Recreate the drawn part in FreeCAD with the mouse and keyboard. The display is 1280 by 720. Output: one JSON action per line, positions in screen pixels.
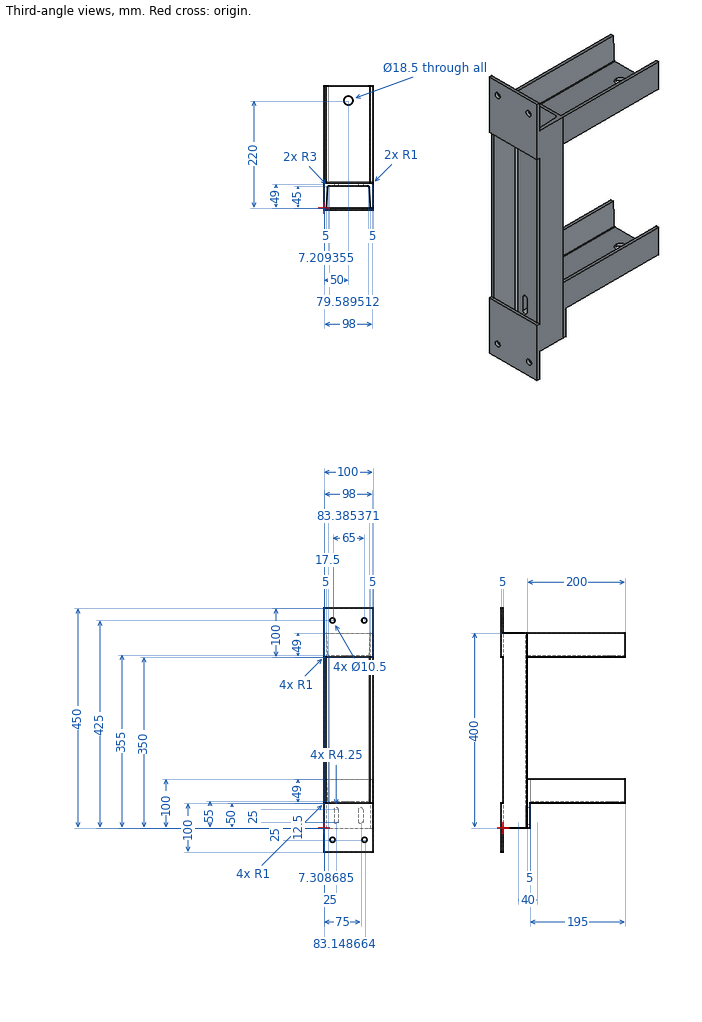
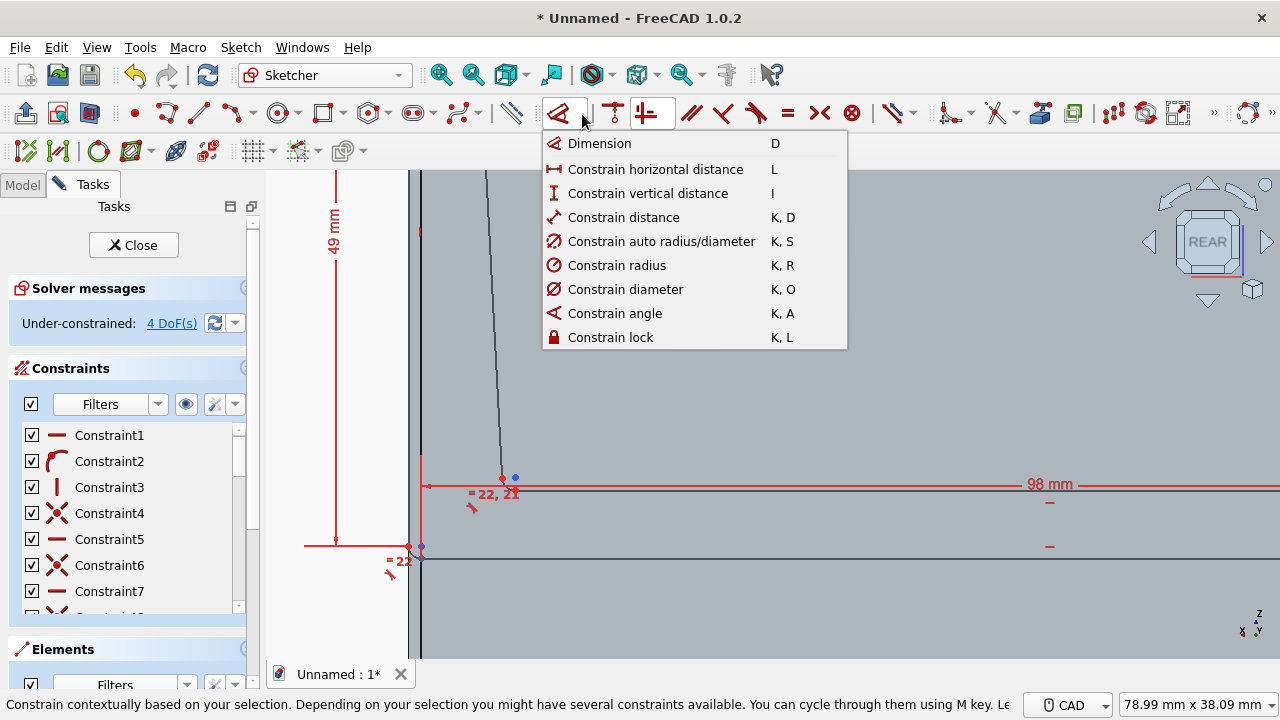
{"action": "left_click", "coordinate": [695, 193]}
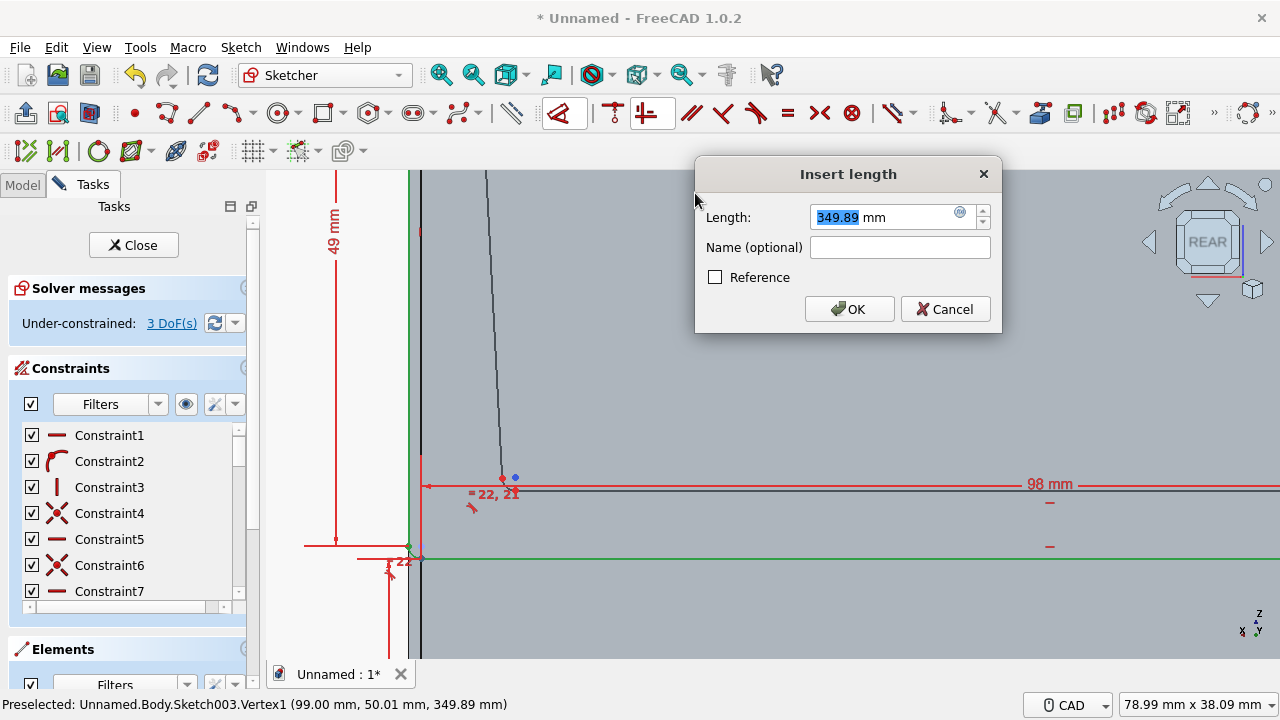
{"action": "type", "text": "350"}
{"action": "key", "text": "Return"}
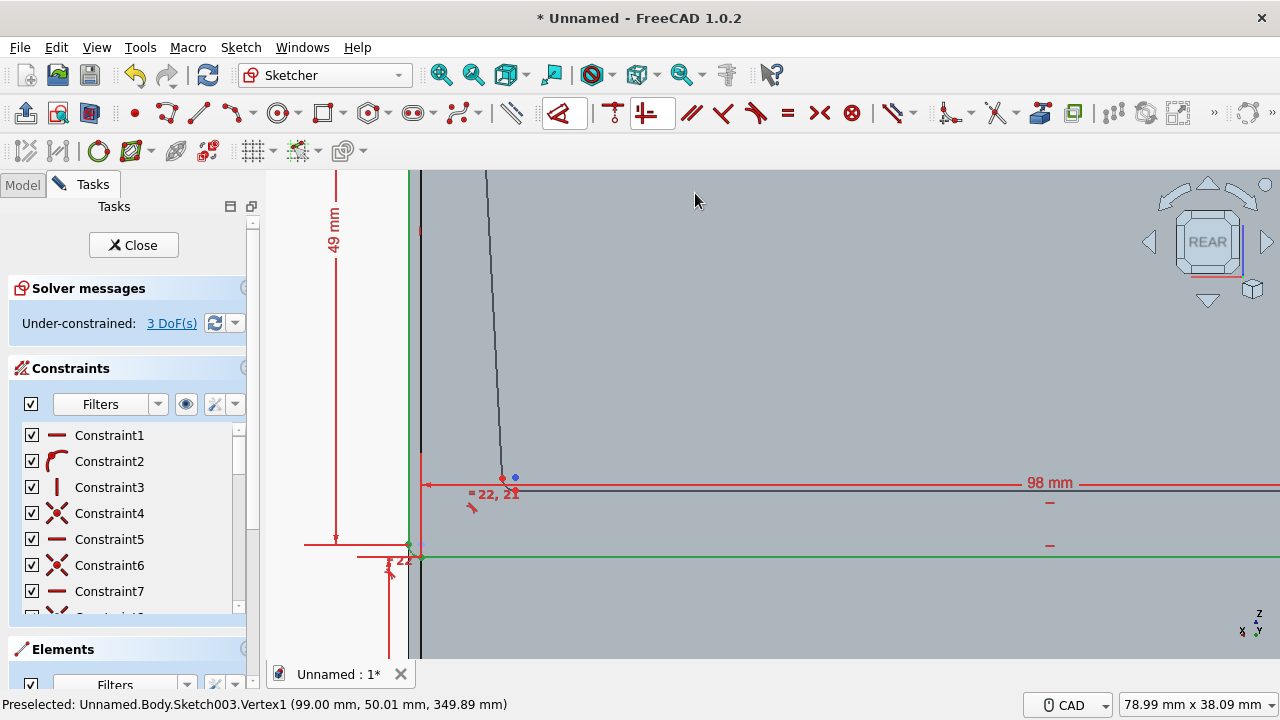
{"action": "scroll", "coordinate": [422, 560], "scroll_direction": "down", "scroll_amount": 4}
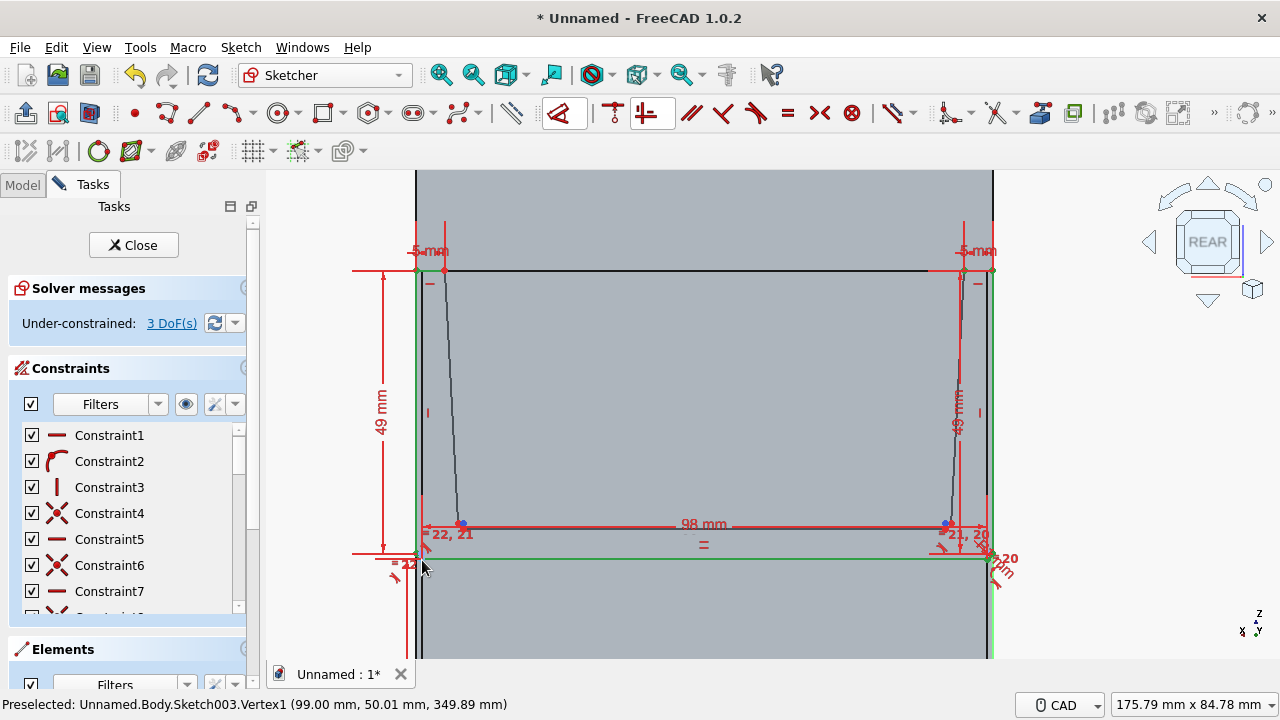
{"action": "scroll", "coordinate": [945, 529], "scroll_direction": "up", "scroll_amount": 4}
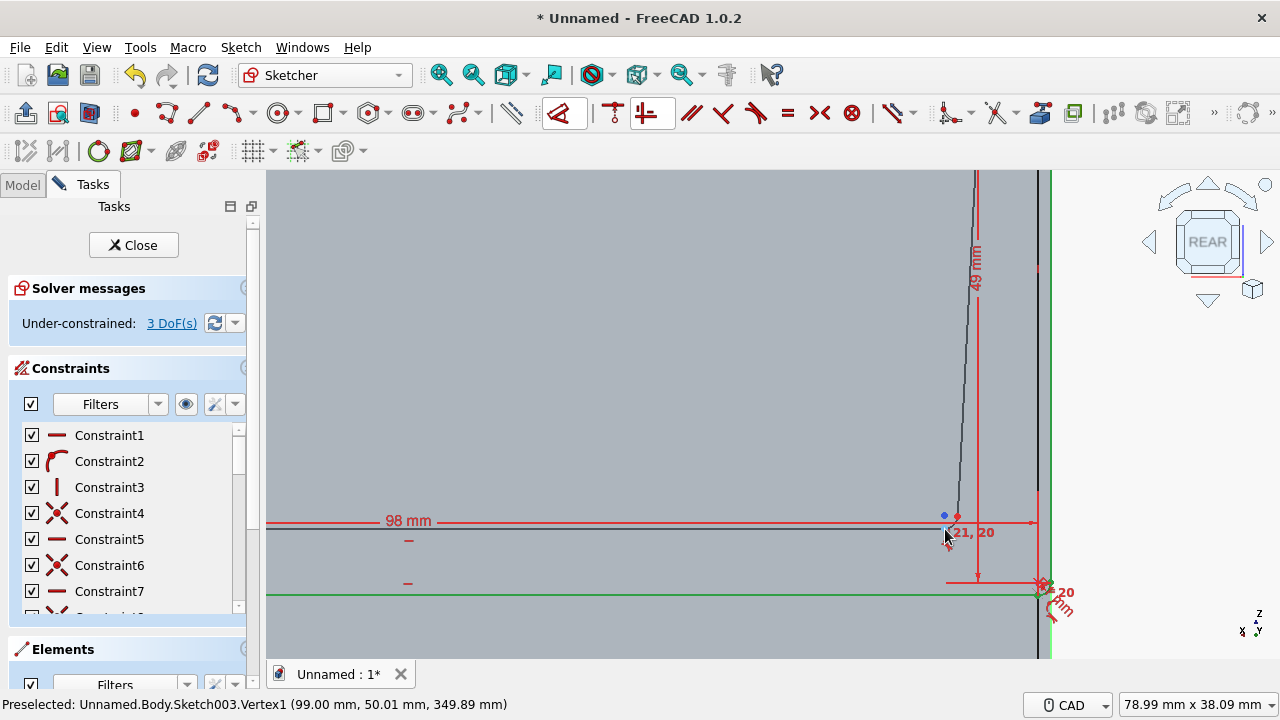
{"action": "left_click", "coordinate": [945, 529]}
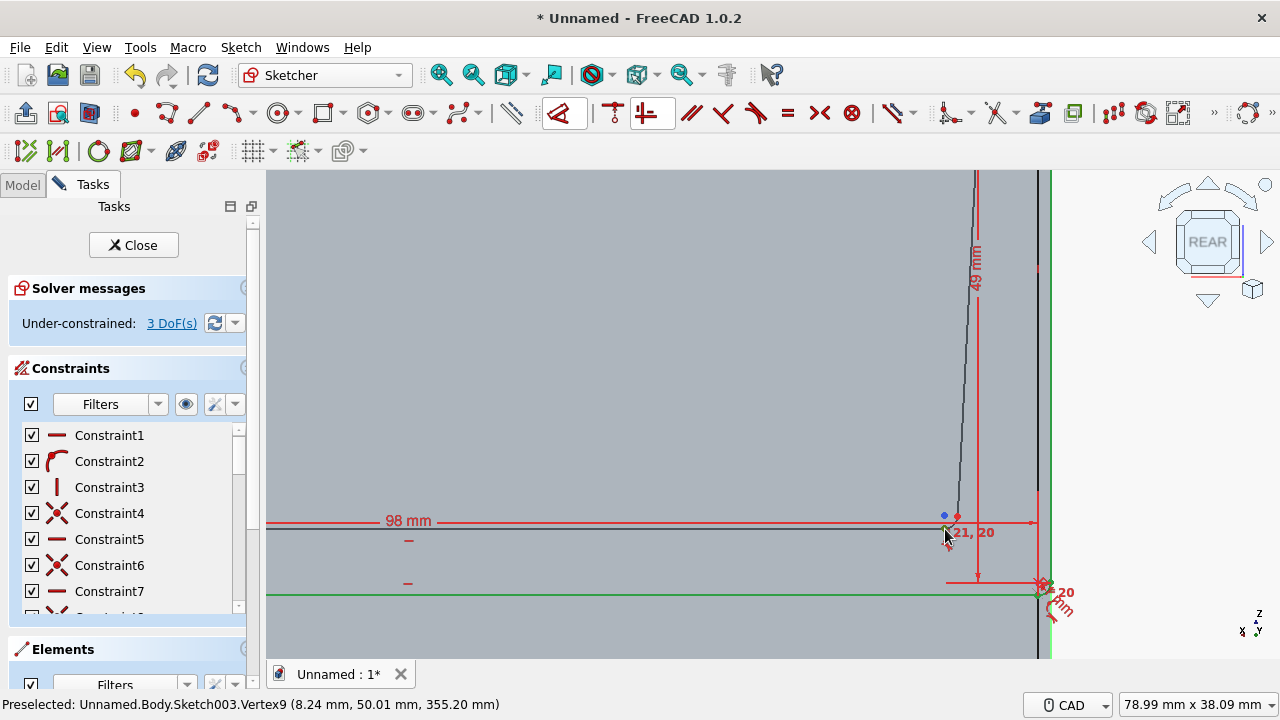
{"action": "left_click", "coordinate": [582, 114]}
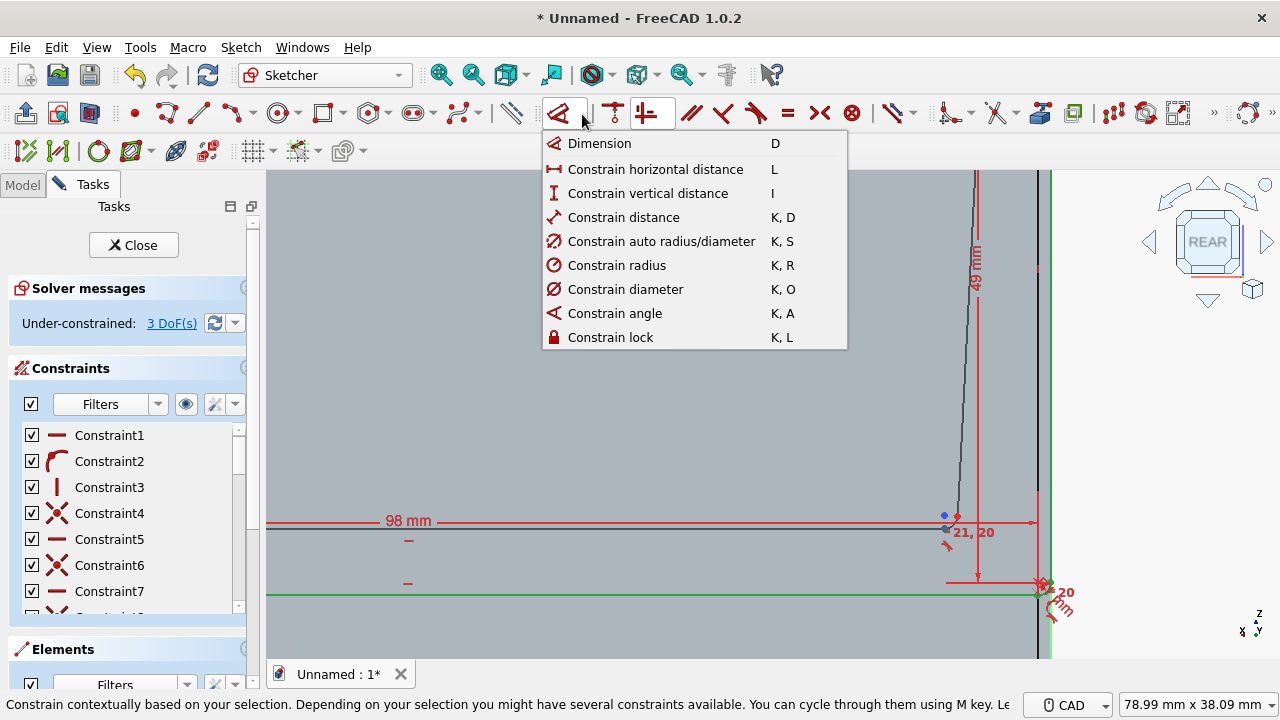
{"action": "left_click", "coordinate": [695, 193]}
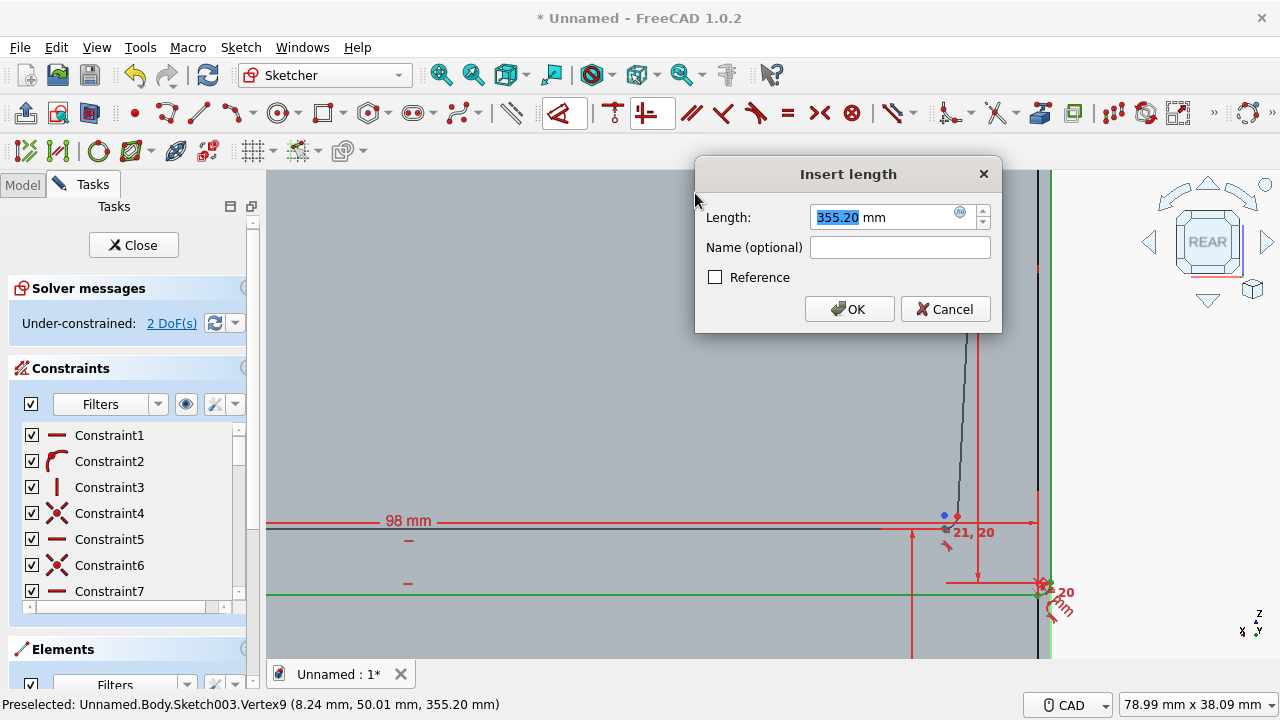
{"action": "type", "text": "355"}
{"action": "key", "text": "Return"}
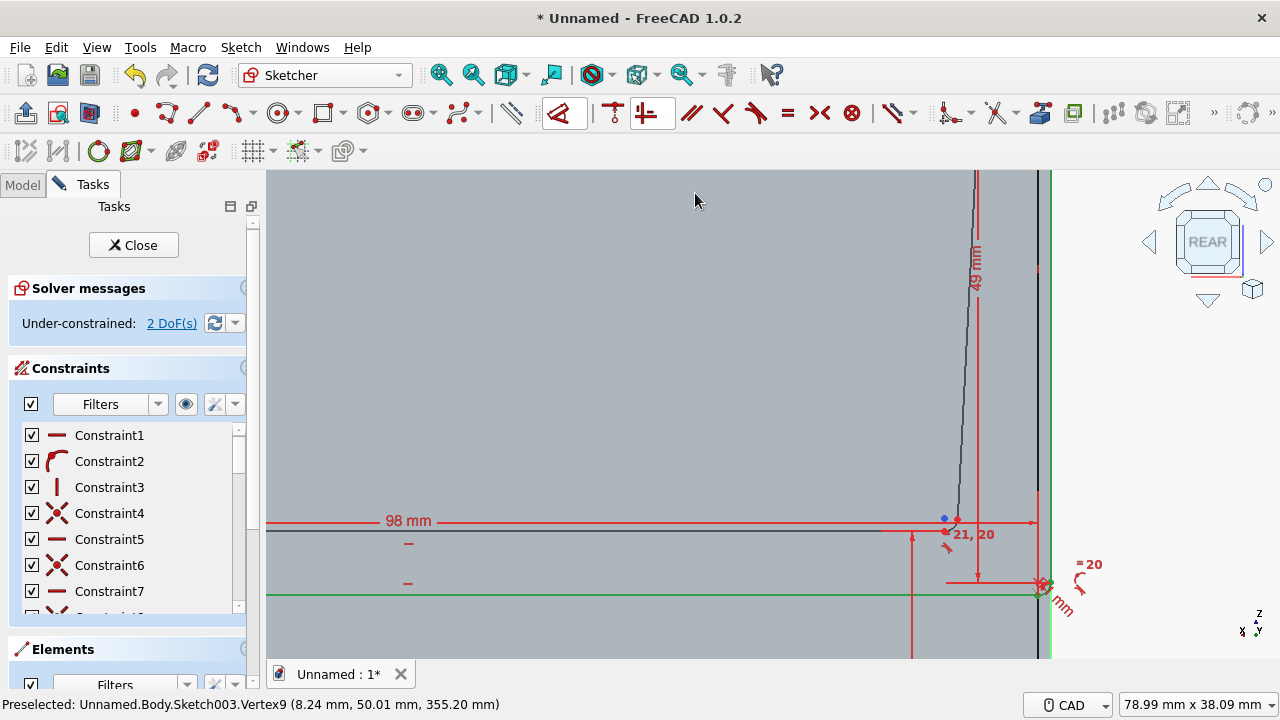
{"action": "left_click", "coordinate": [623, 531]}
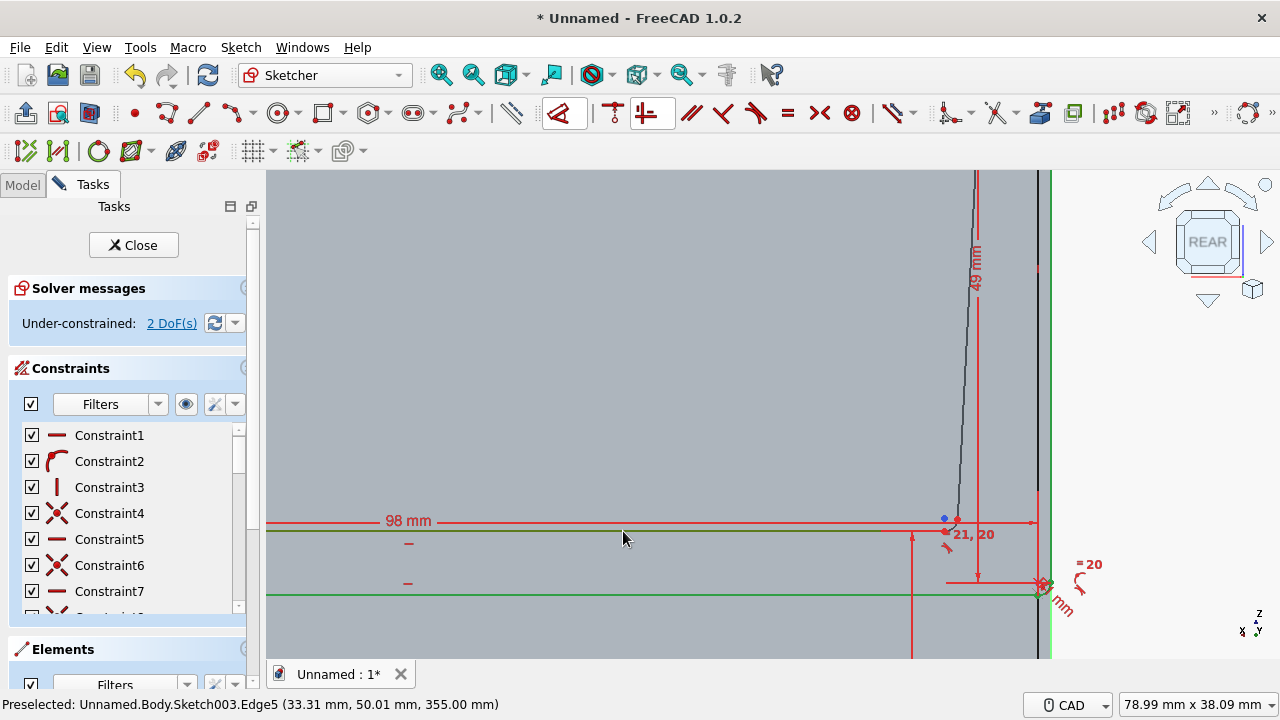
{"action": "key", "text": "l"}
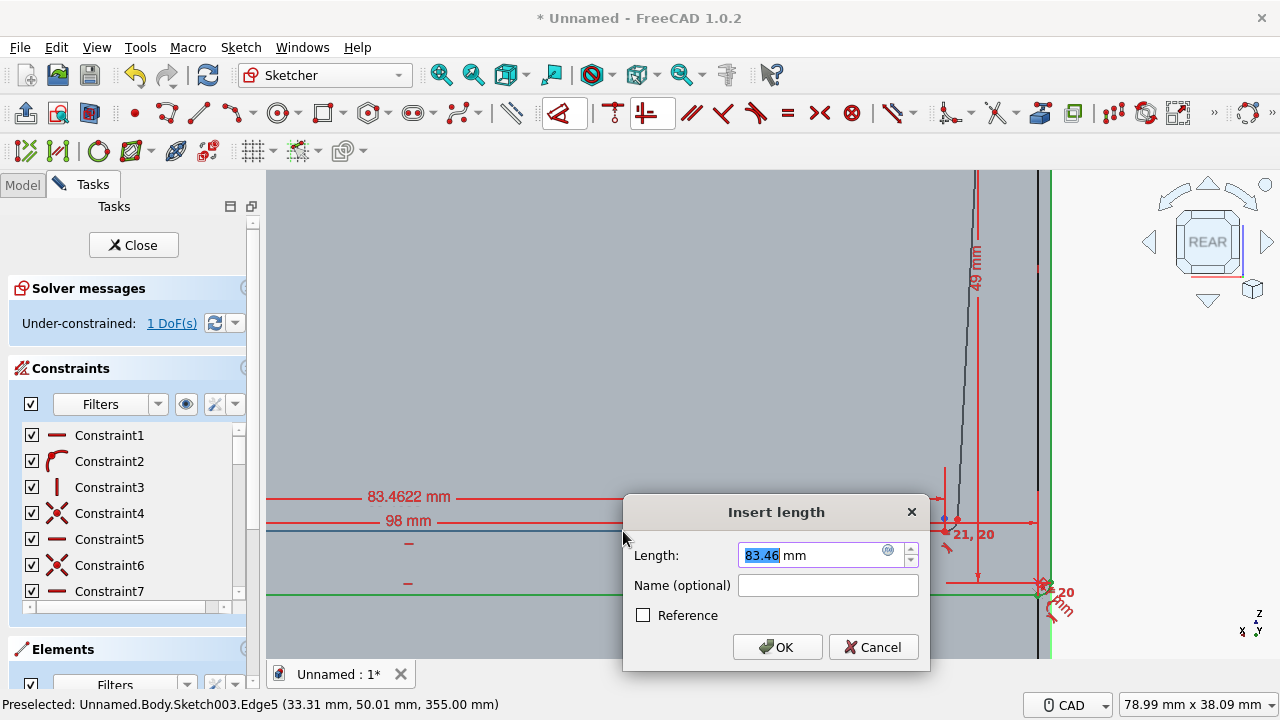
{"action": "type", "text": "83.385371"}
{"action": "key", "text": "Return"}